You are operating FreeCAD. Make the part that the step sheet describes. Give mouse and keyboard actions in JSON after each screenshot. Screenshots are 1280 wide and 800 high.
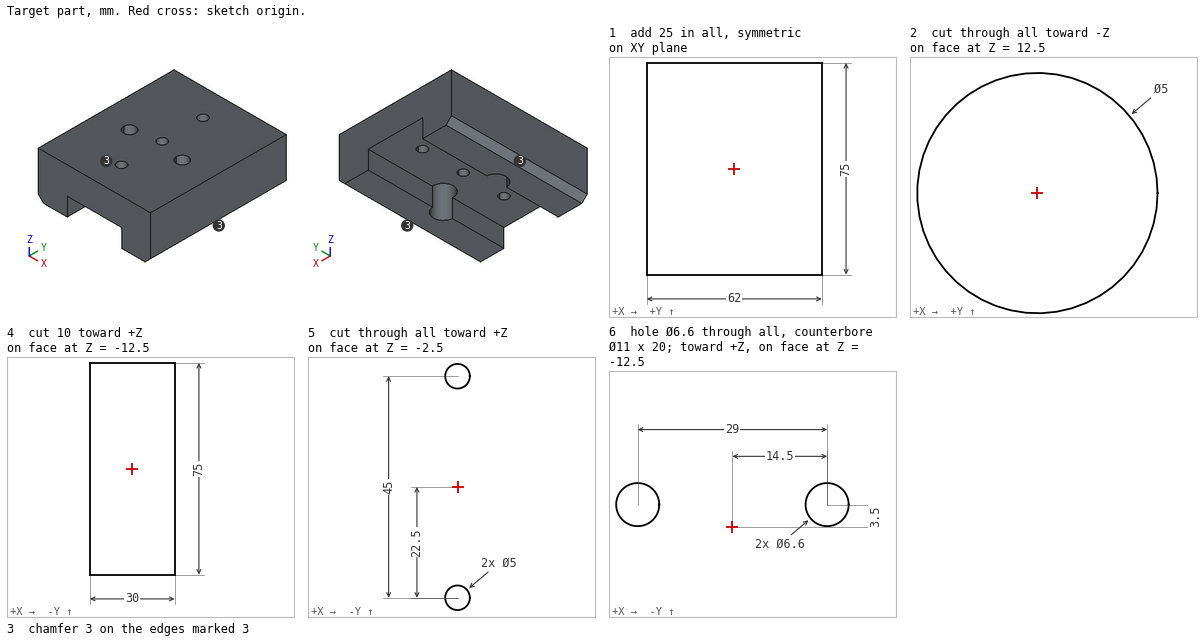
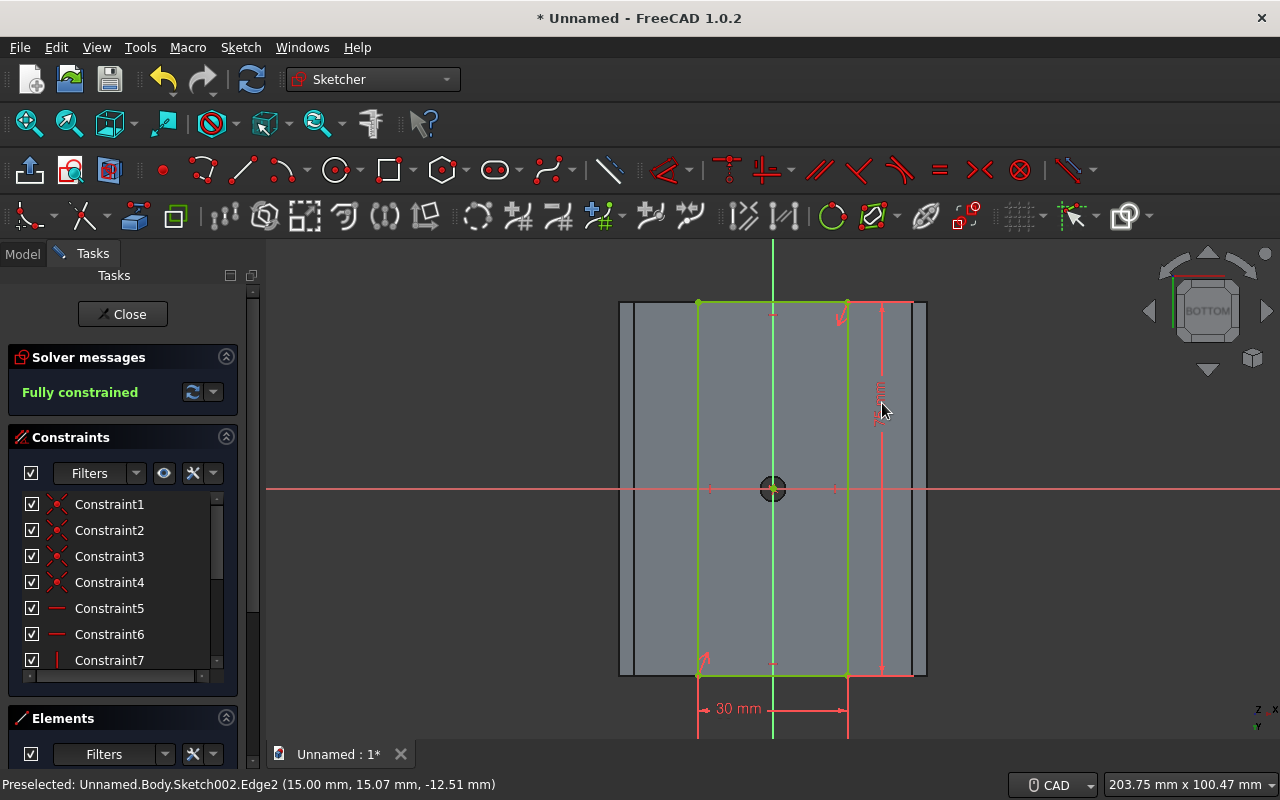
{"action": "left_click", "coordinate": [123, 314]}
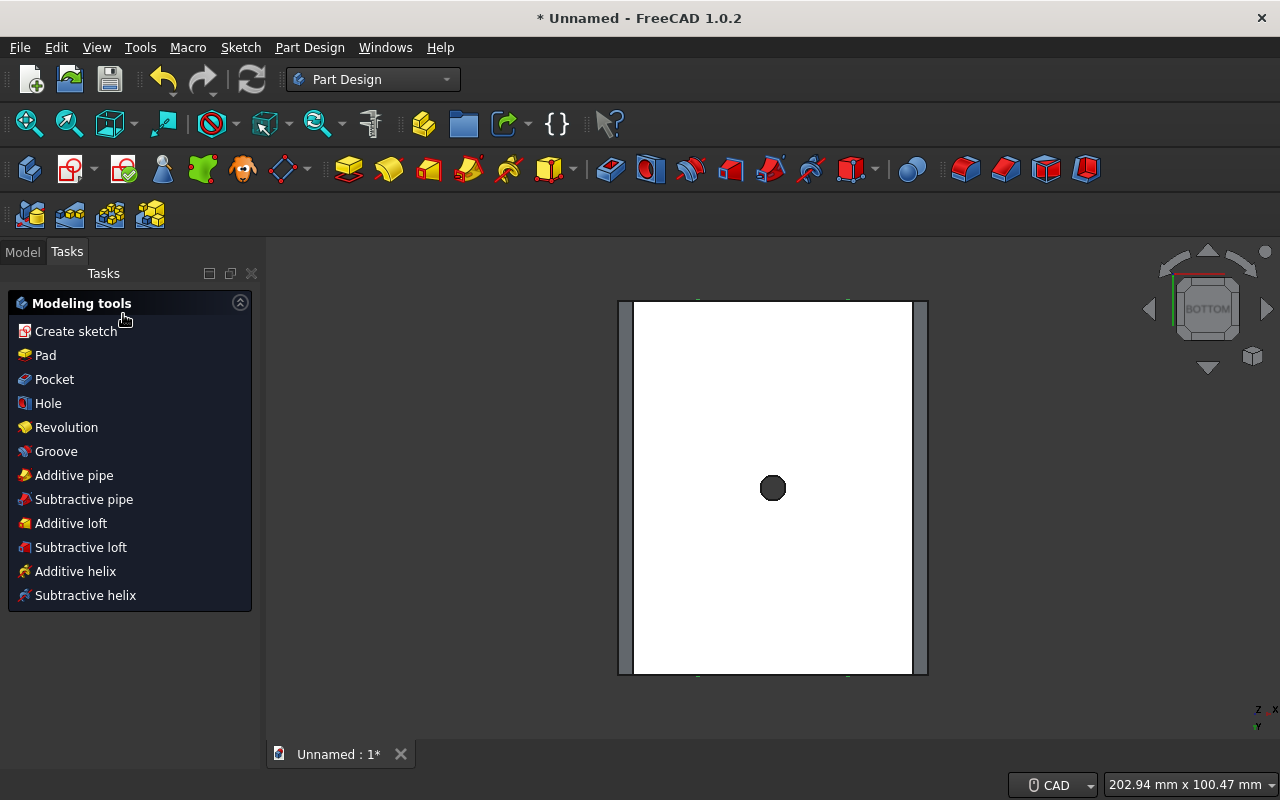
{"action": "left_click", "coordinate": [612, 170]}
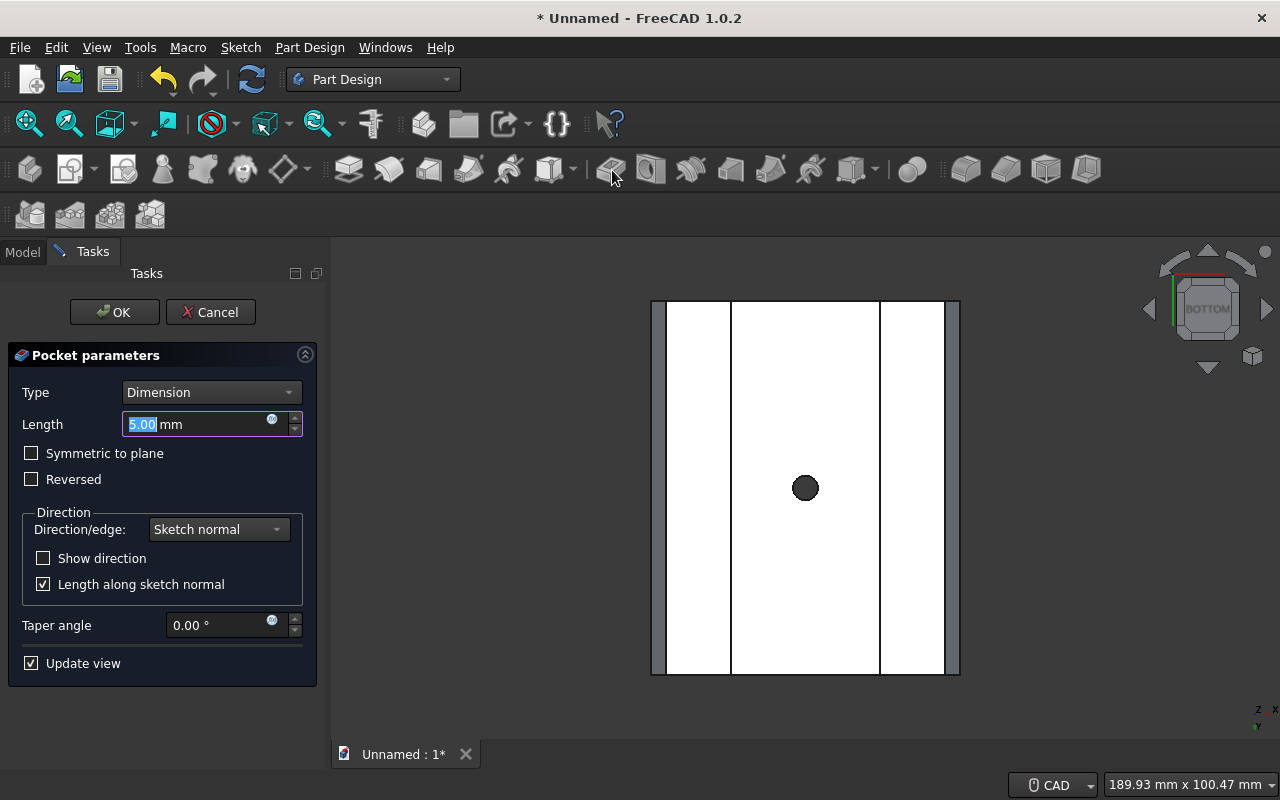
{"action": "type", "text": "10"}
{"action": "key", "text": "Tab"}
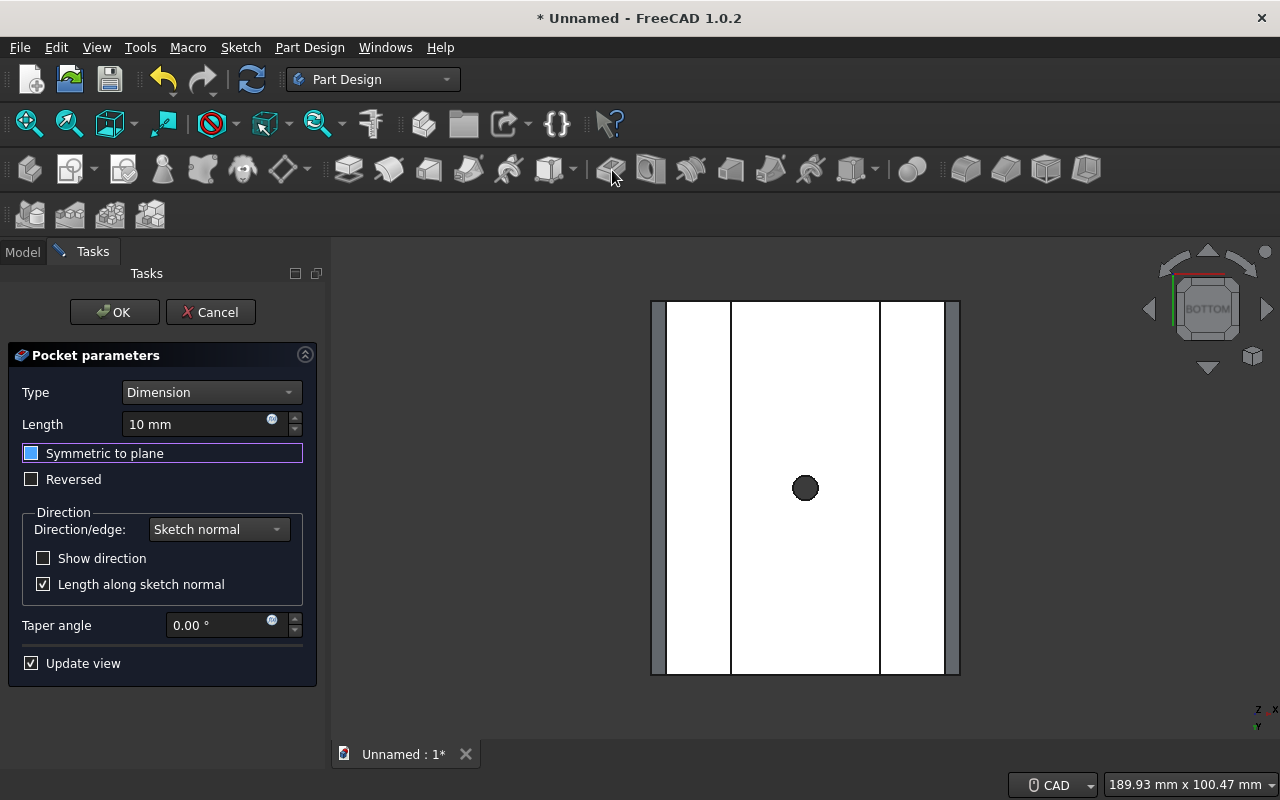
{"action": "left_click", "coordinate": [115, 312]}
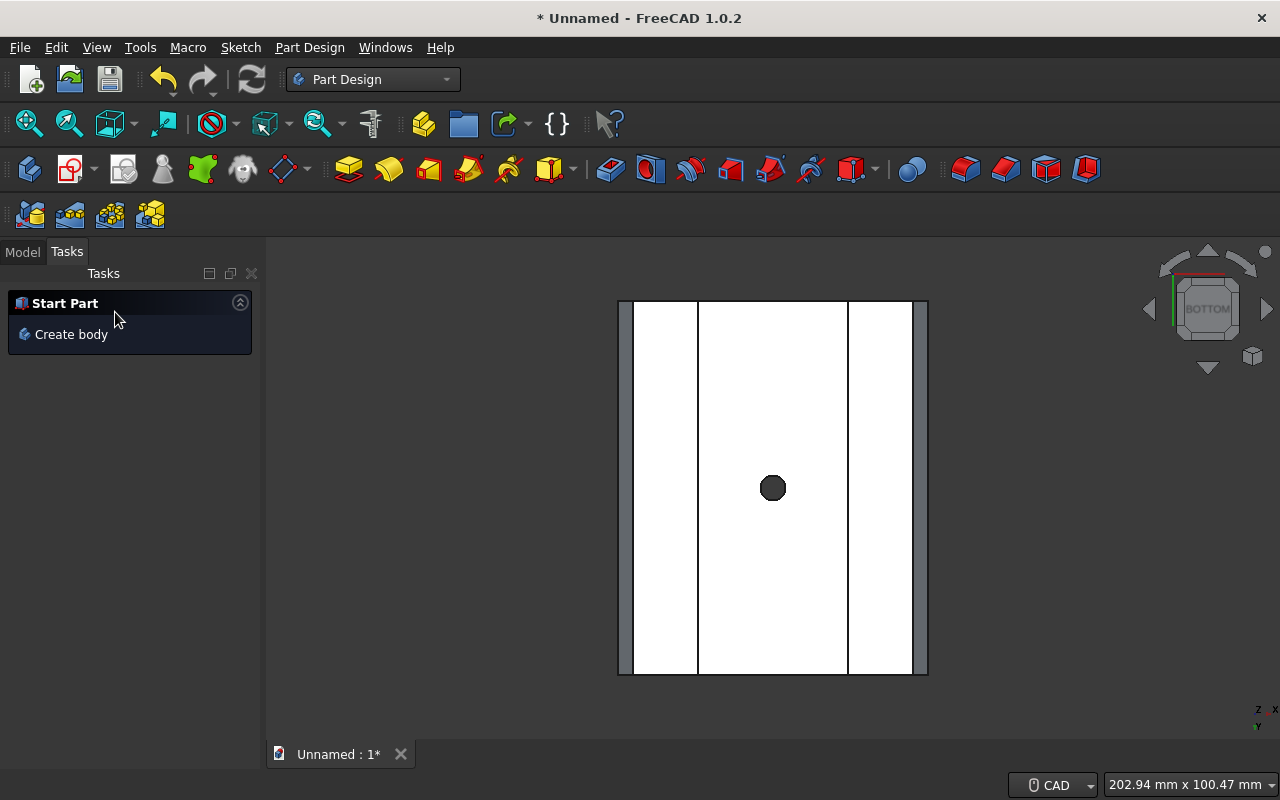
{"action": "left_click", "coordinate": [773, 594]}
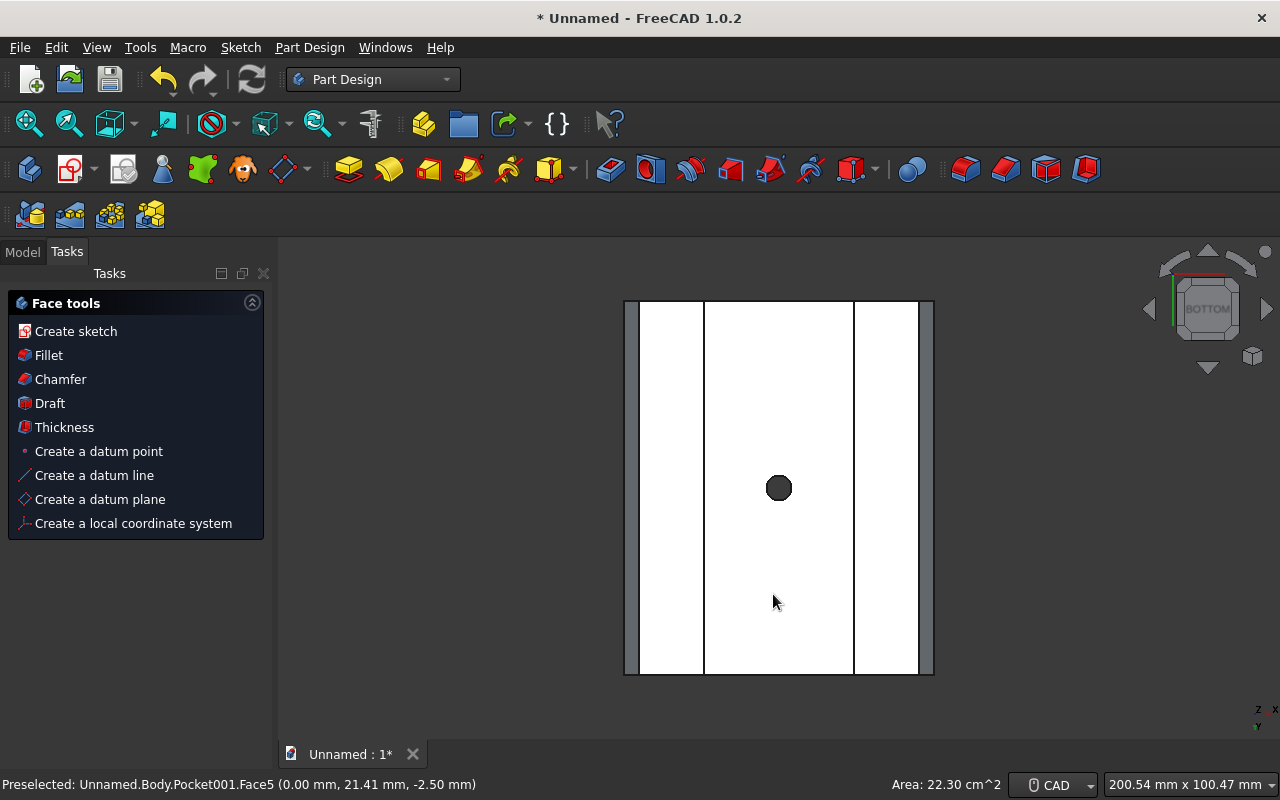
{"action": "left_click", "coordinate": [70, 170]}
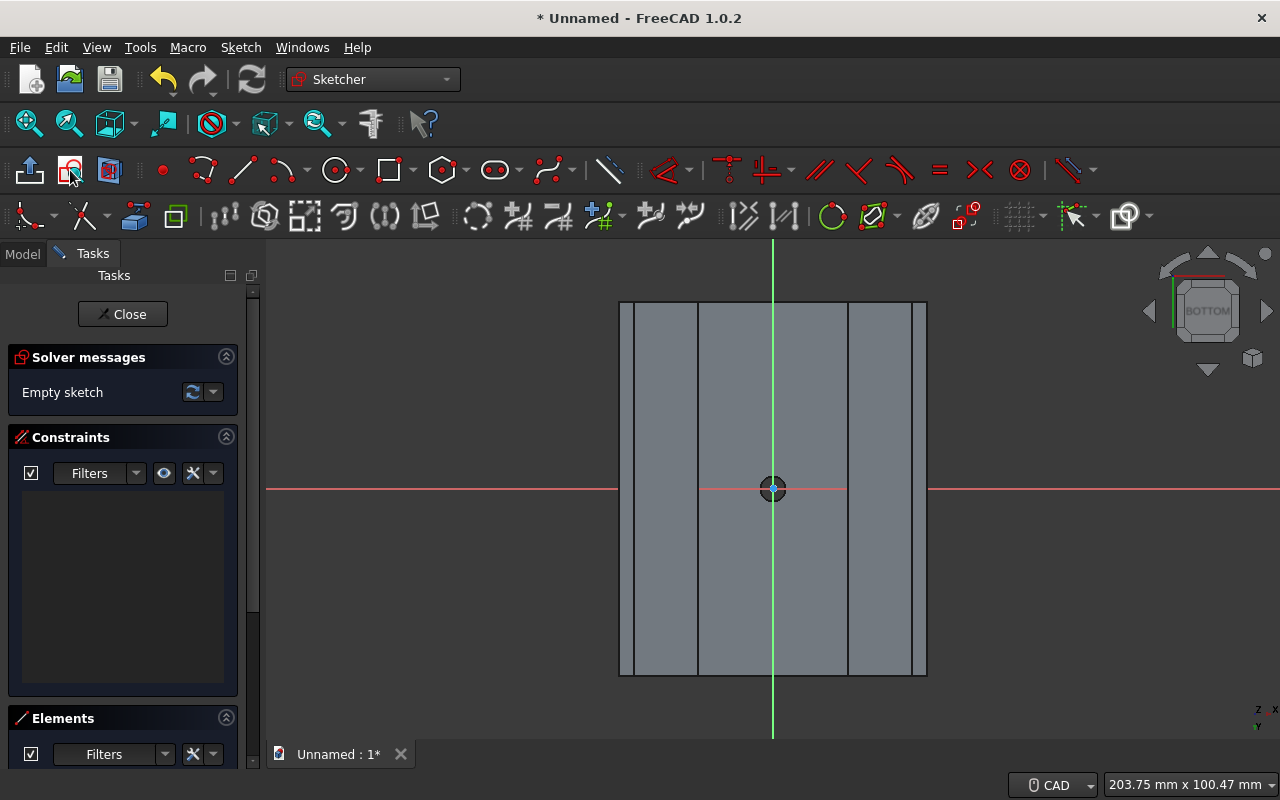
{"action": "key", "text": "g c"}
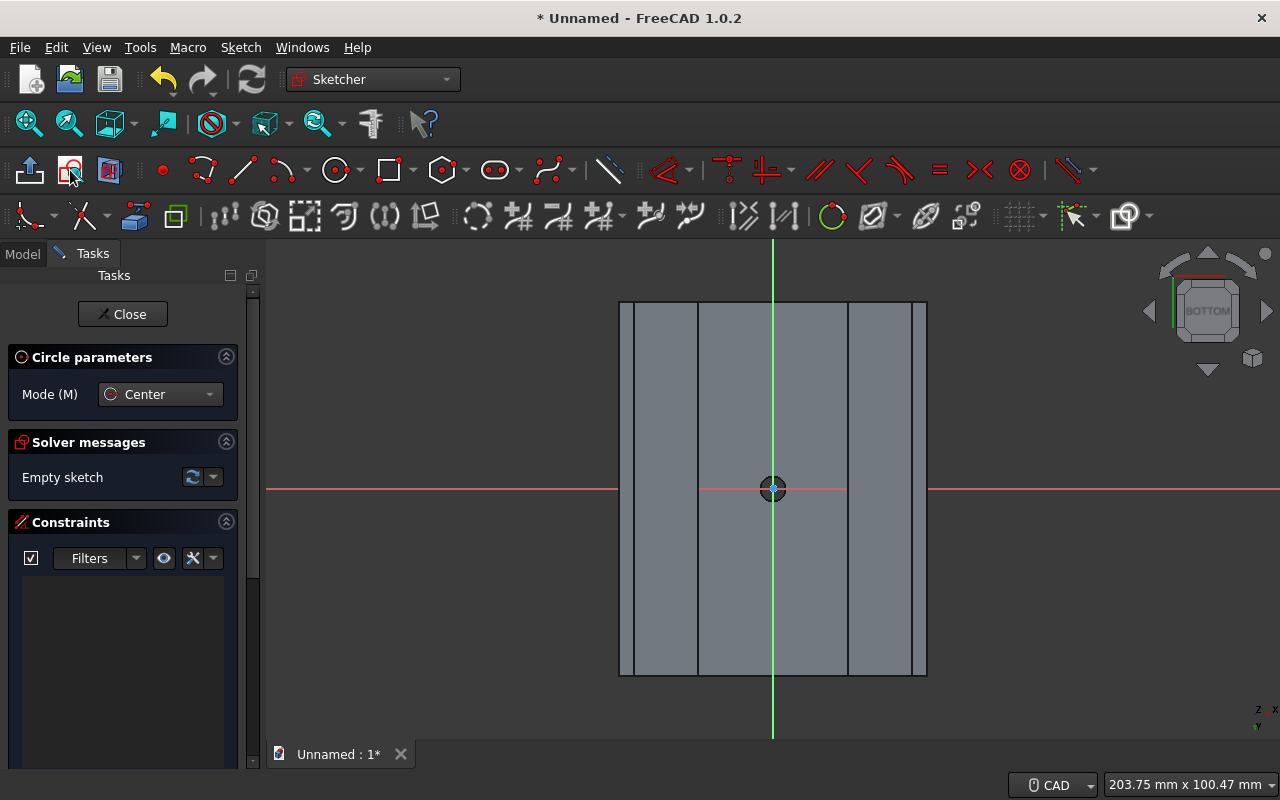
{"action": "scroll", "coordinate": [773, 601], "scroll_direction": "up", "scroll_amount": 4}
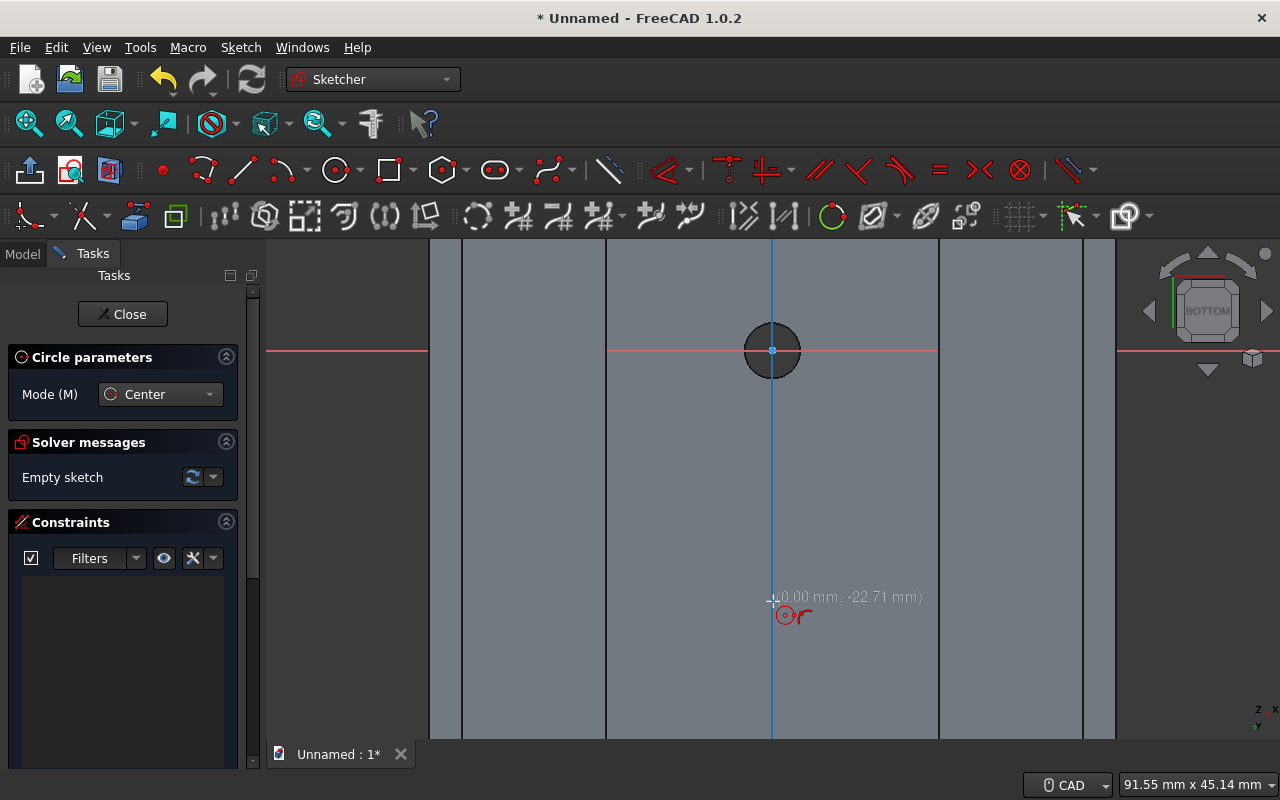
{"action": "left_click", "coordinate": [772, 600]}
{"action": "left_click", "coordinate": [792, 580]}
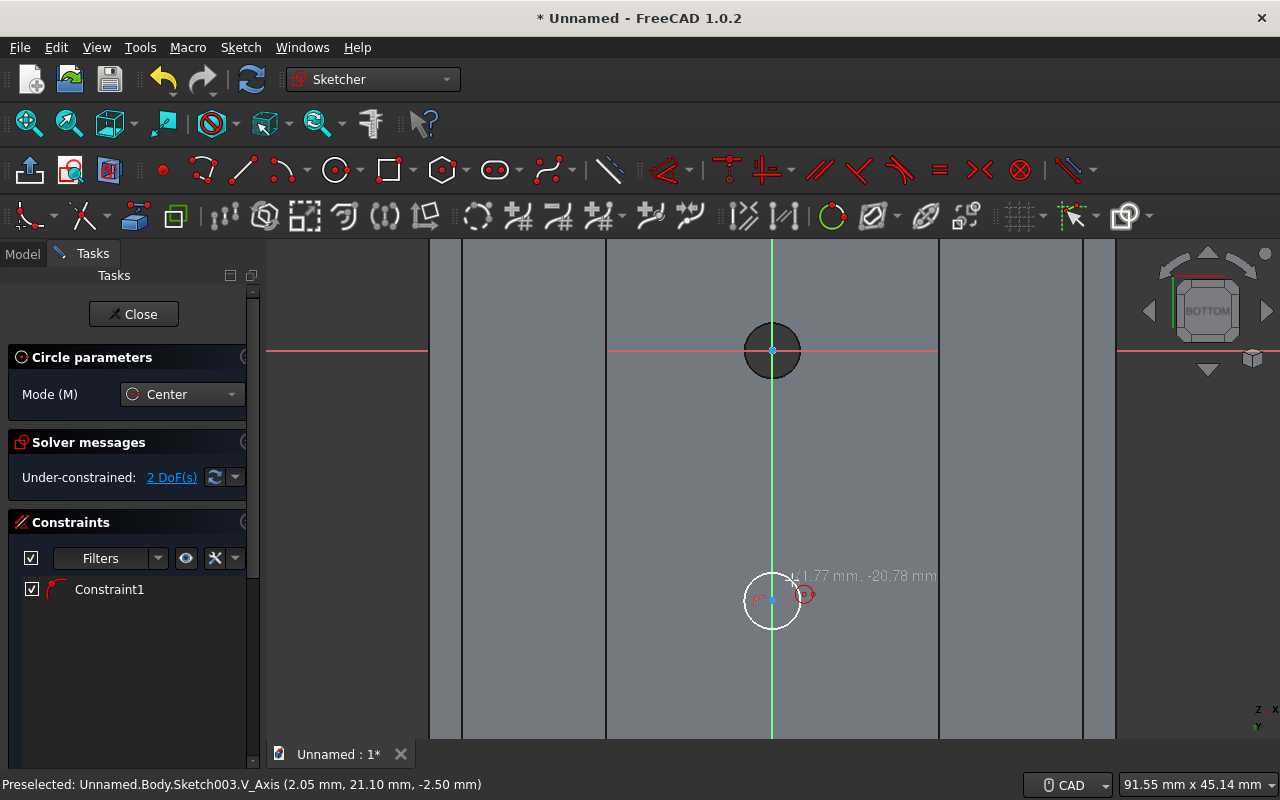
{"action": "scroll", "coordinate": [622, 657], "scroll_direction": "down", "scroll_amount": 3}